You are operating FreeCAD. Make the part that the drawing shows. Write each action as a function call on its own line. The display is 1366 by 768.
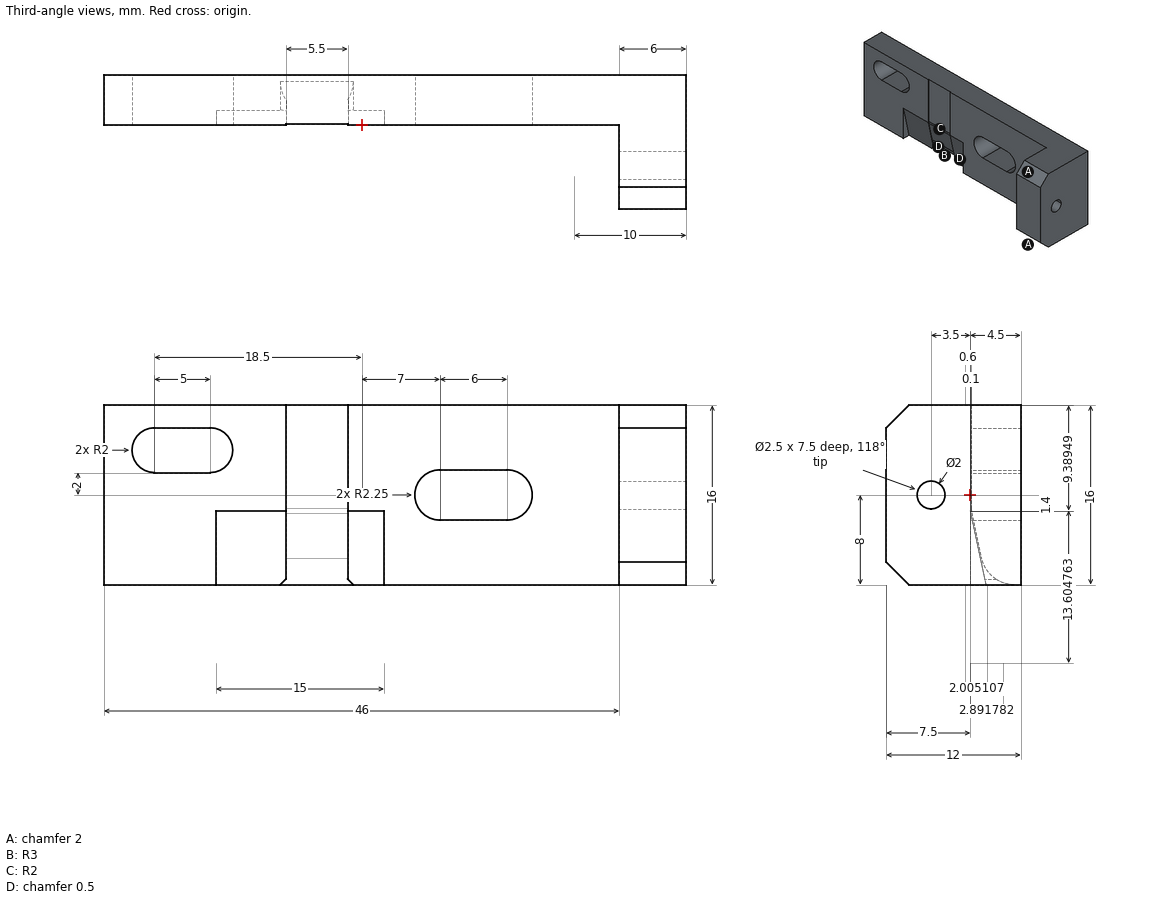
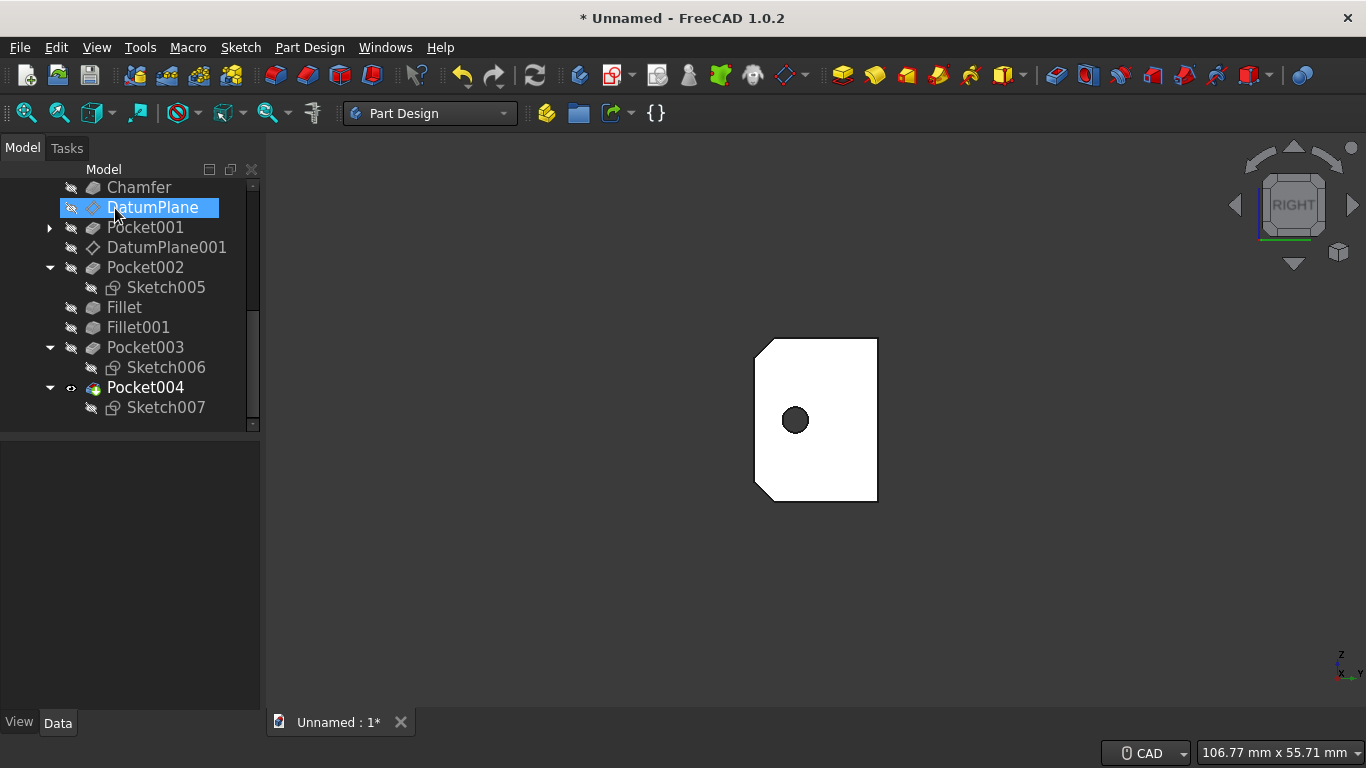
click(28, 114)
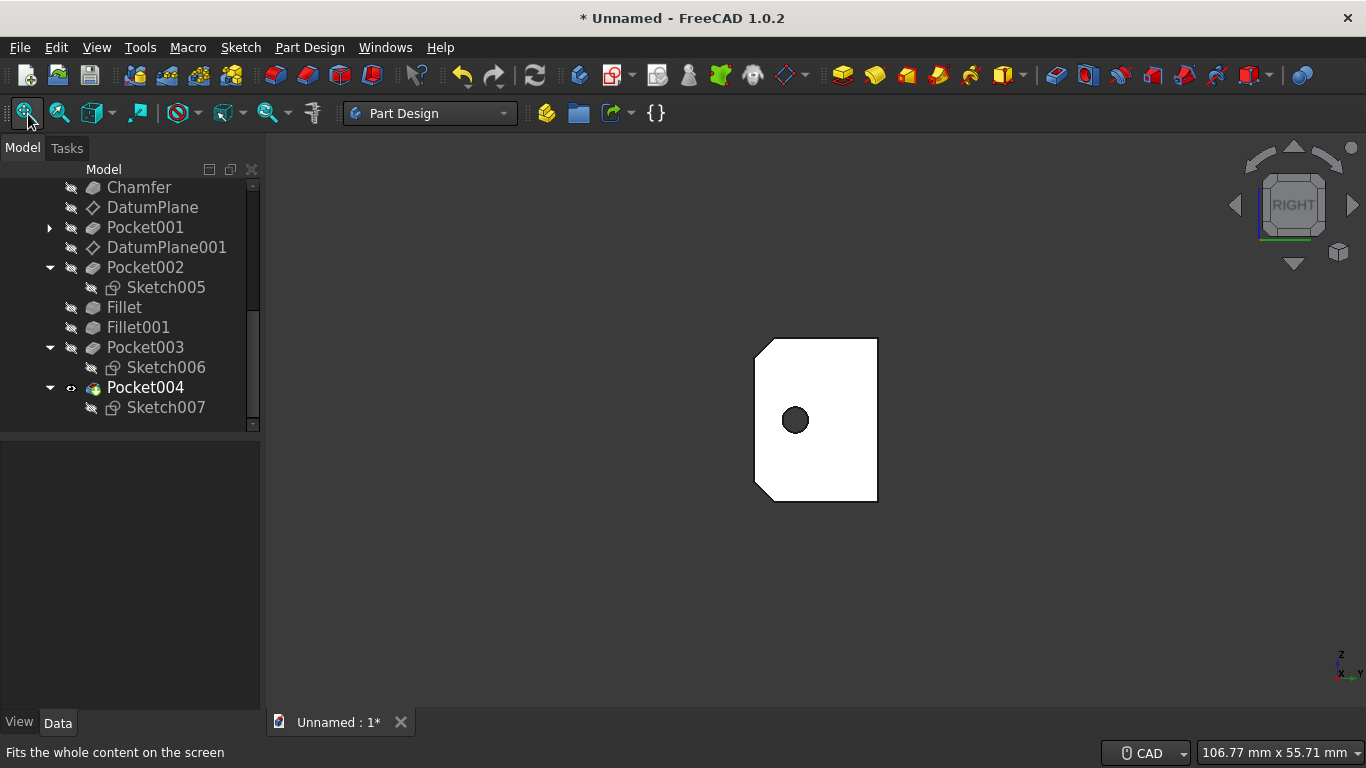
key(5)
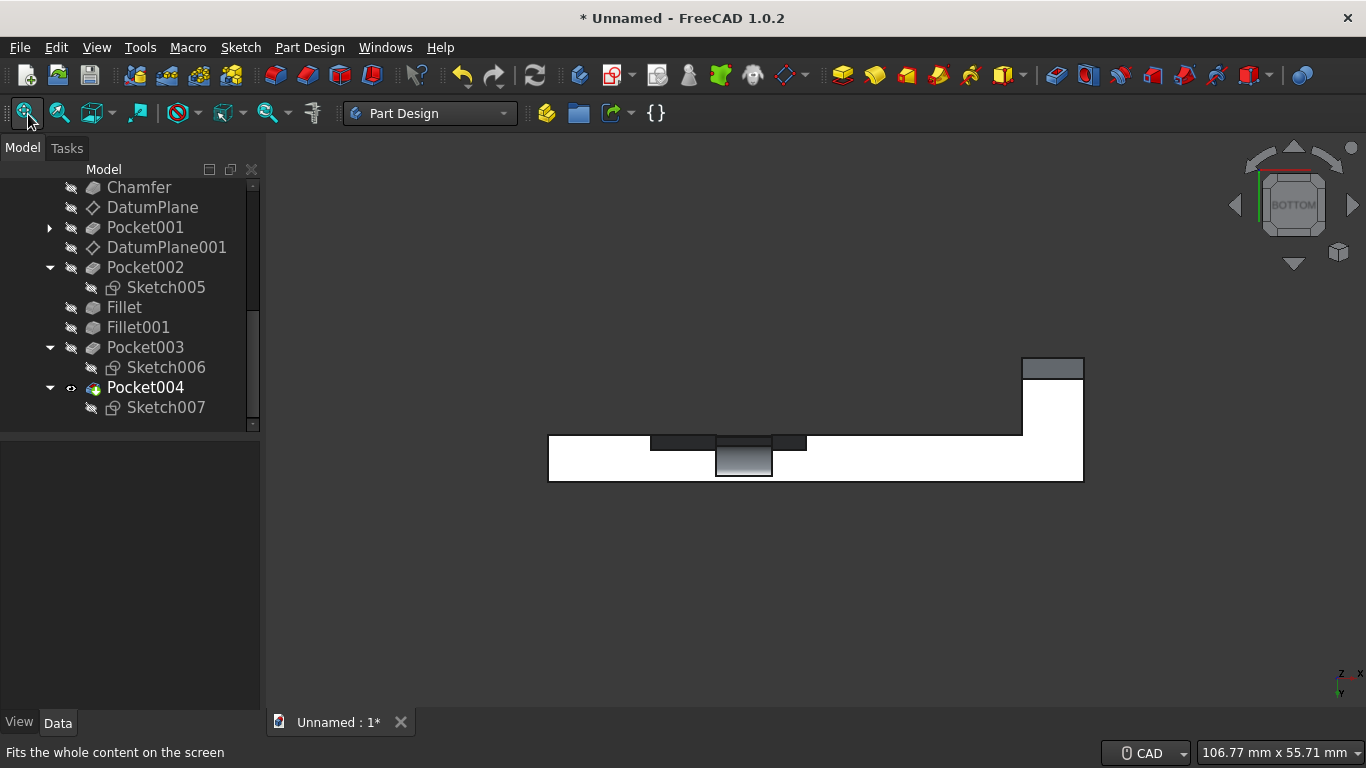
click(772, 462)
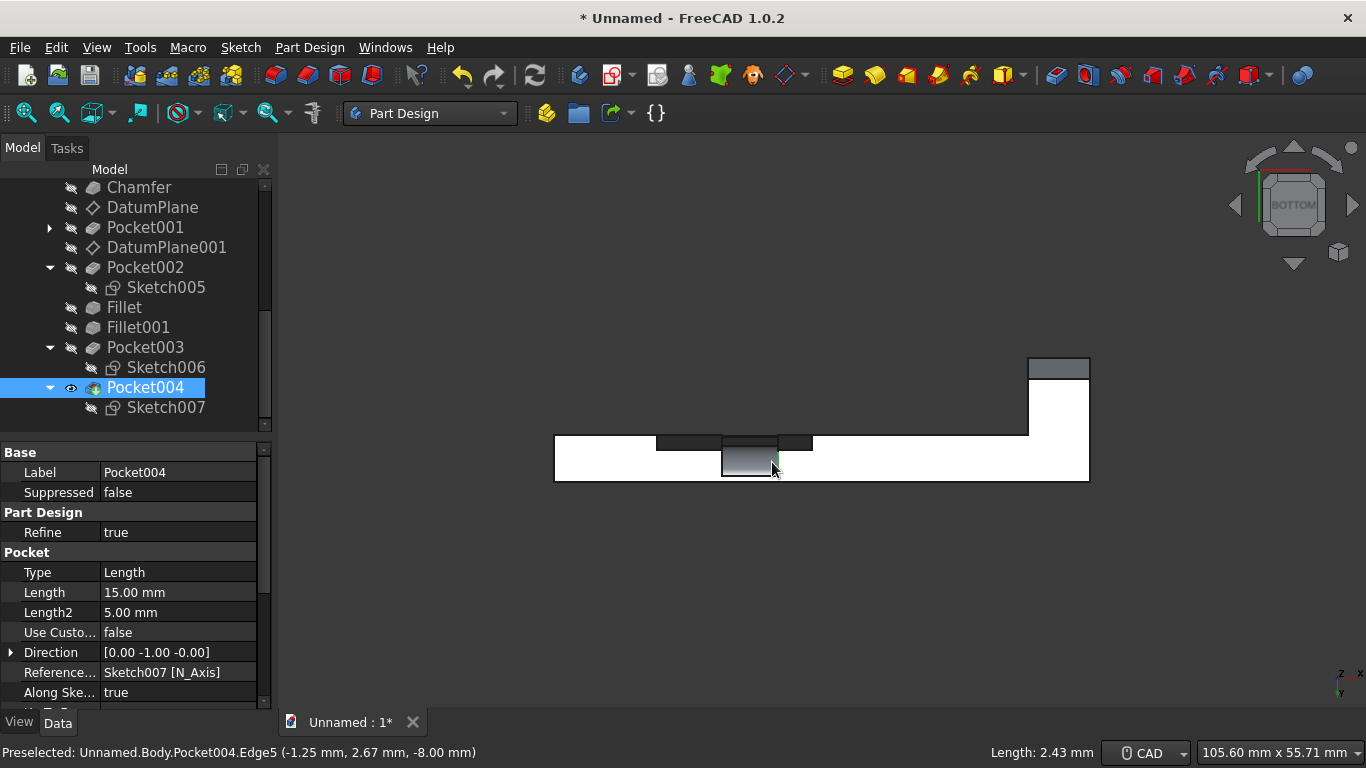
click(722, 462, ctrl)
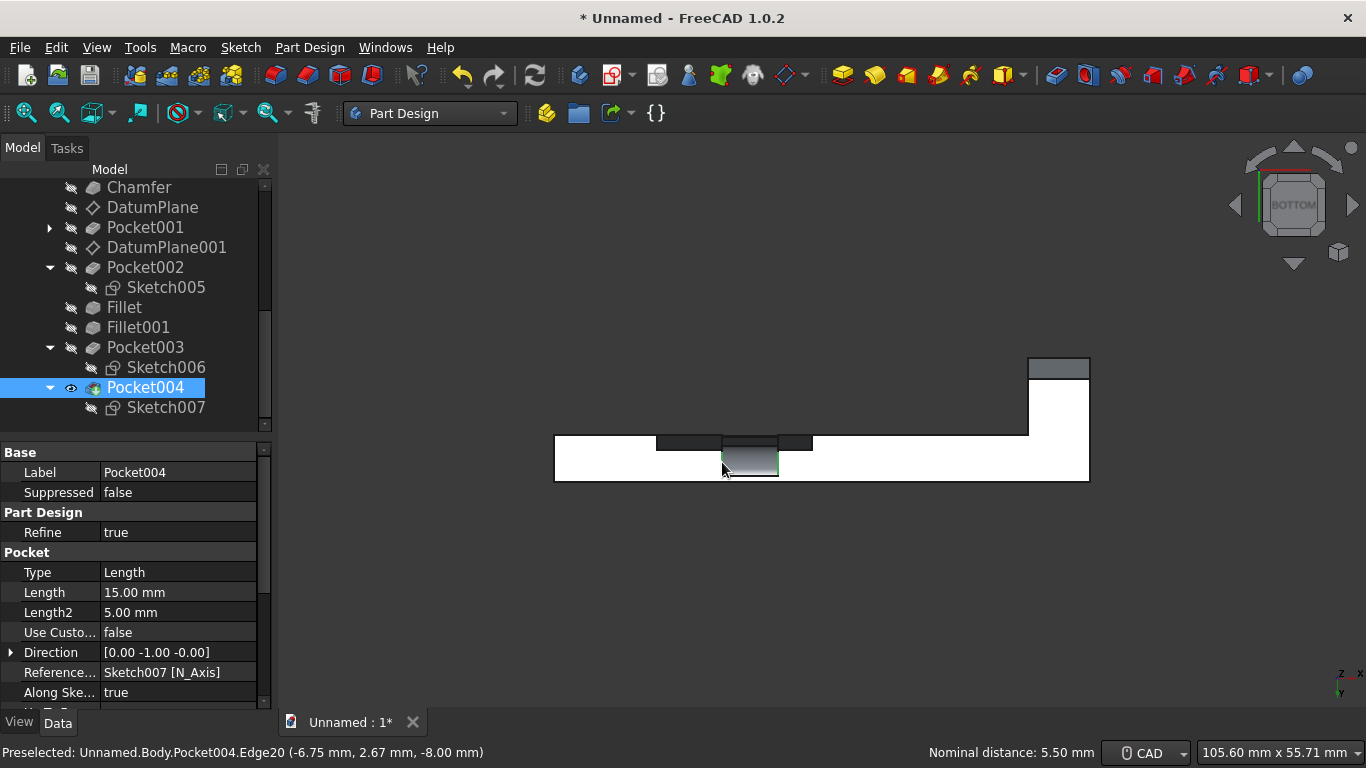
click(308, 76)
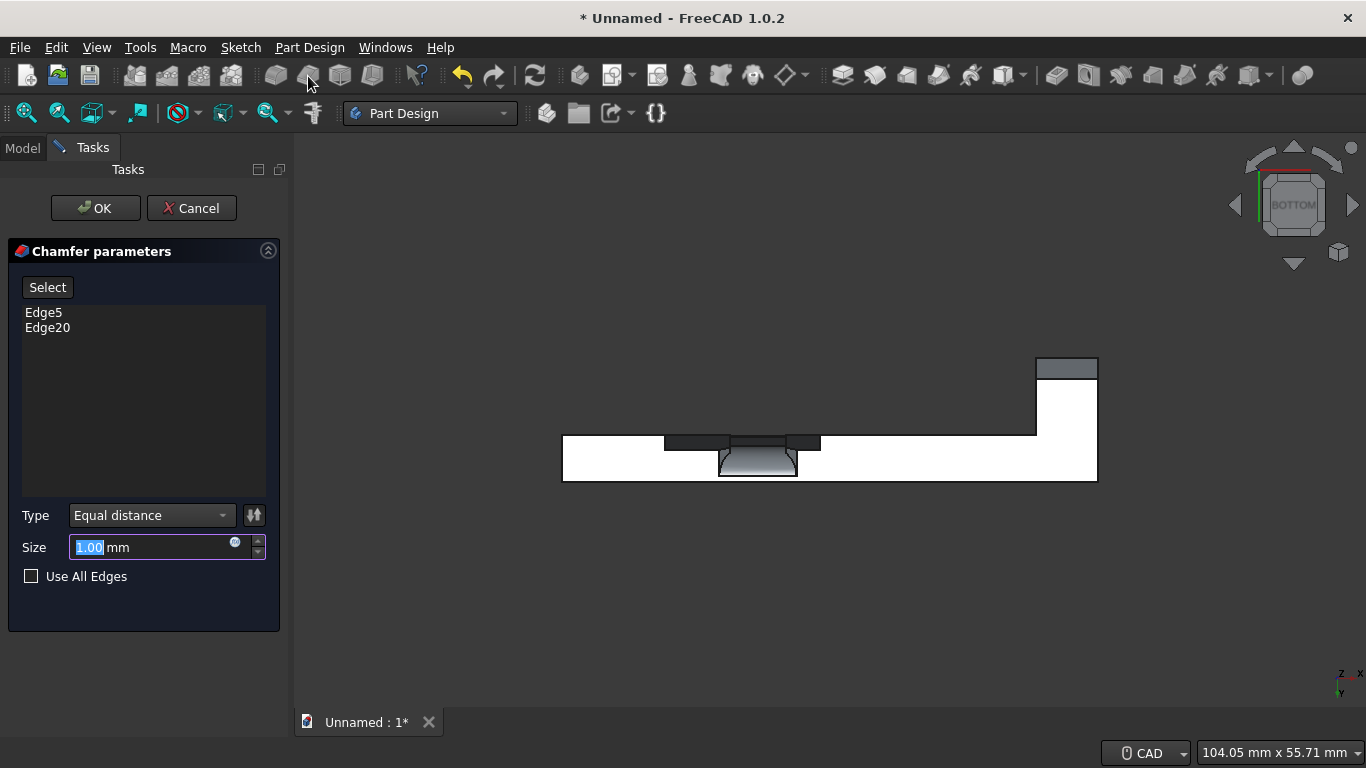
text(0.5)
key(Tab)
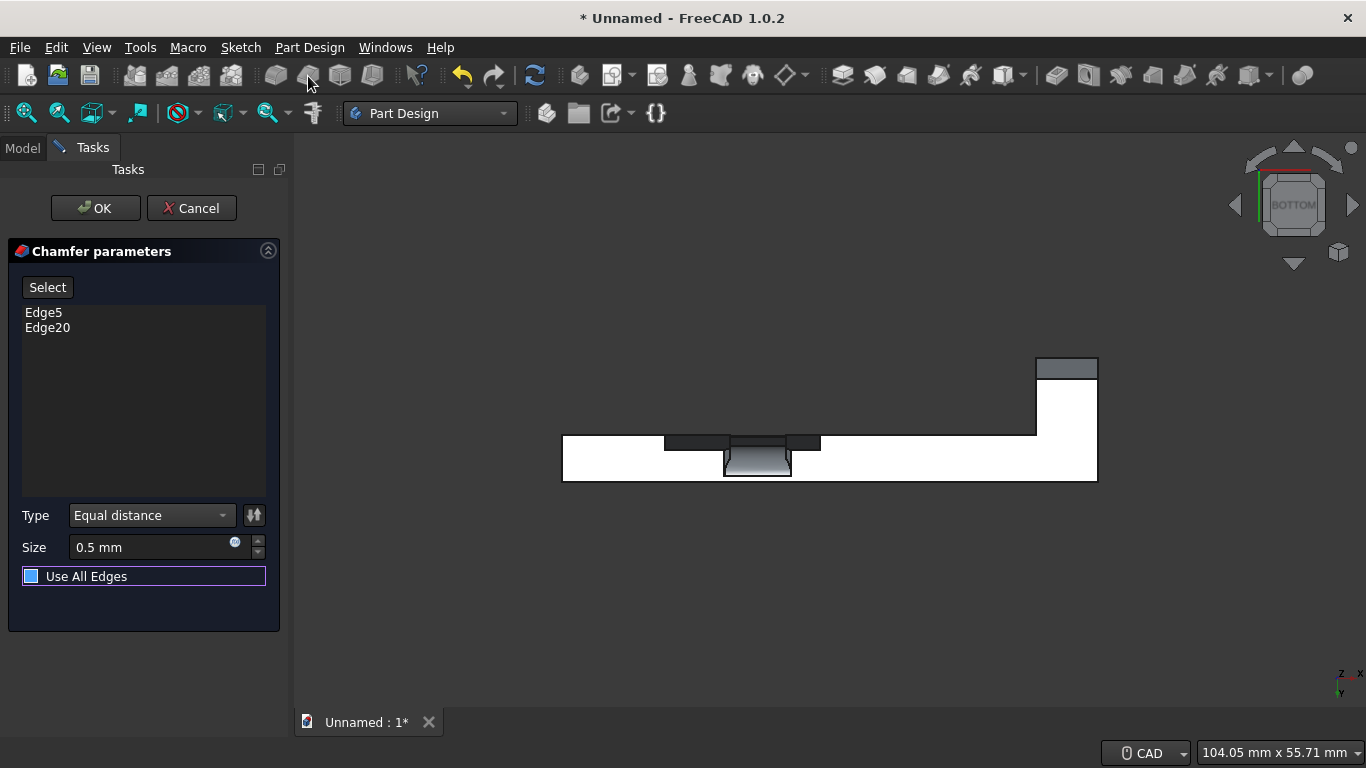
click(96, 208)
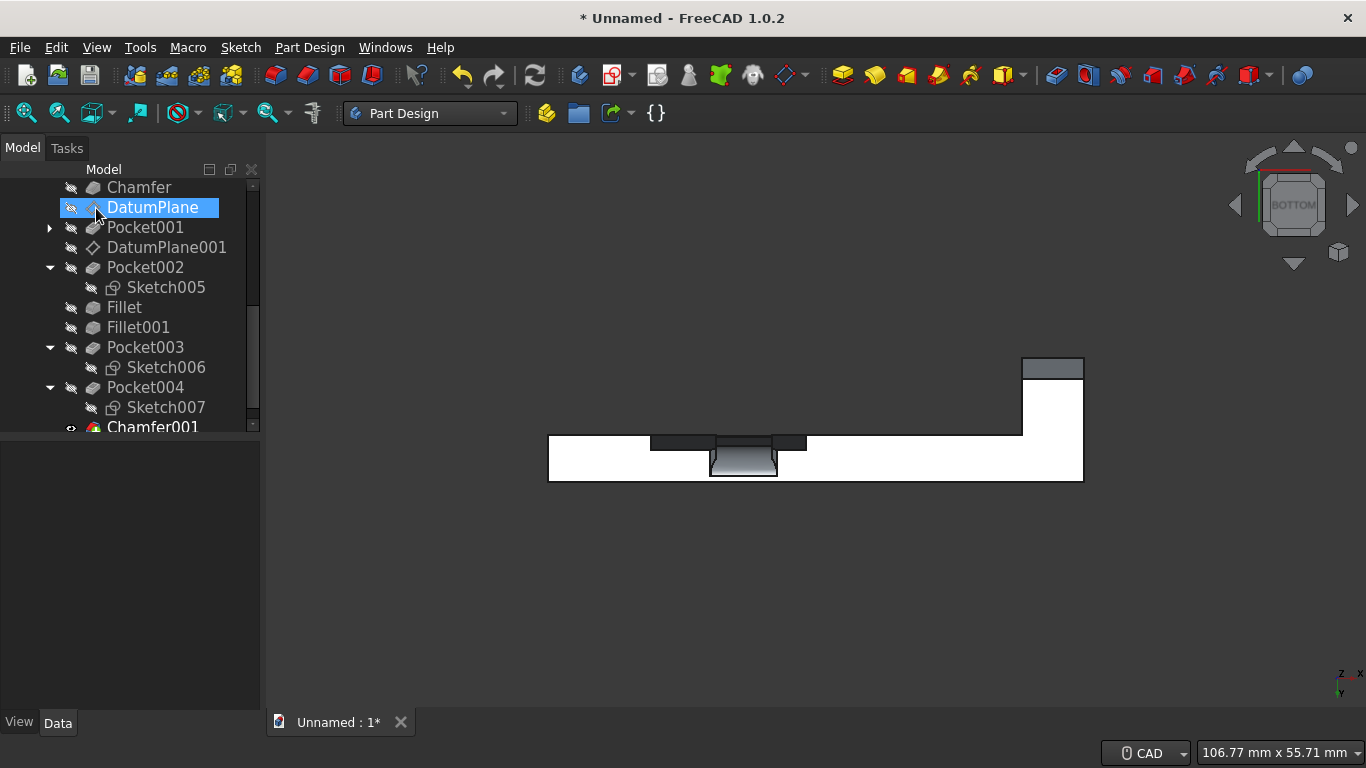
key(0)